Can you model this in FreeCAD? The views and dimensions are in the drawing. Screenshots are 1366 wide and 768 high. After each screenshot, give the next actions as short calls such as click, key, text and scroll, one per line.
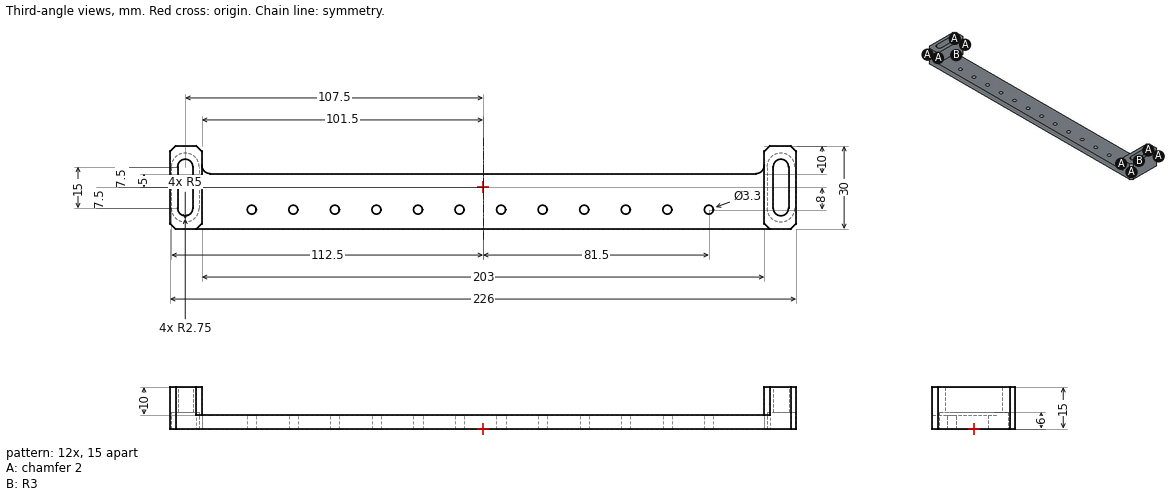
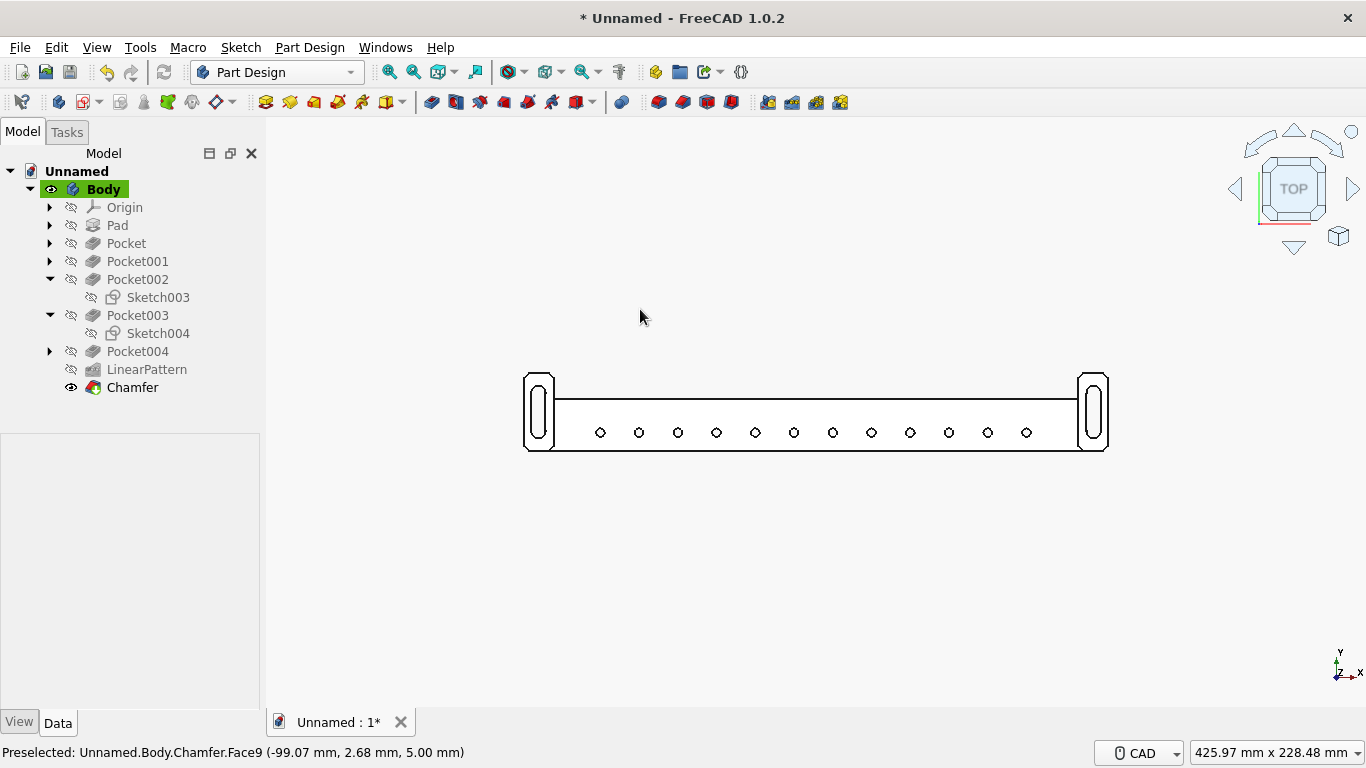
scroll(554, 398, up, 6)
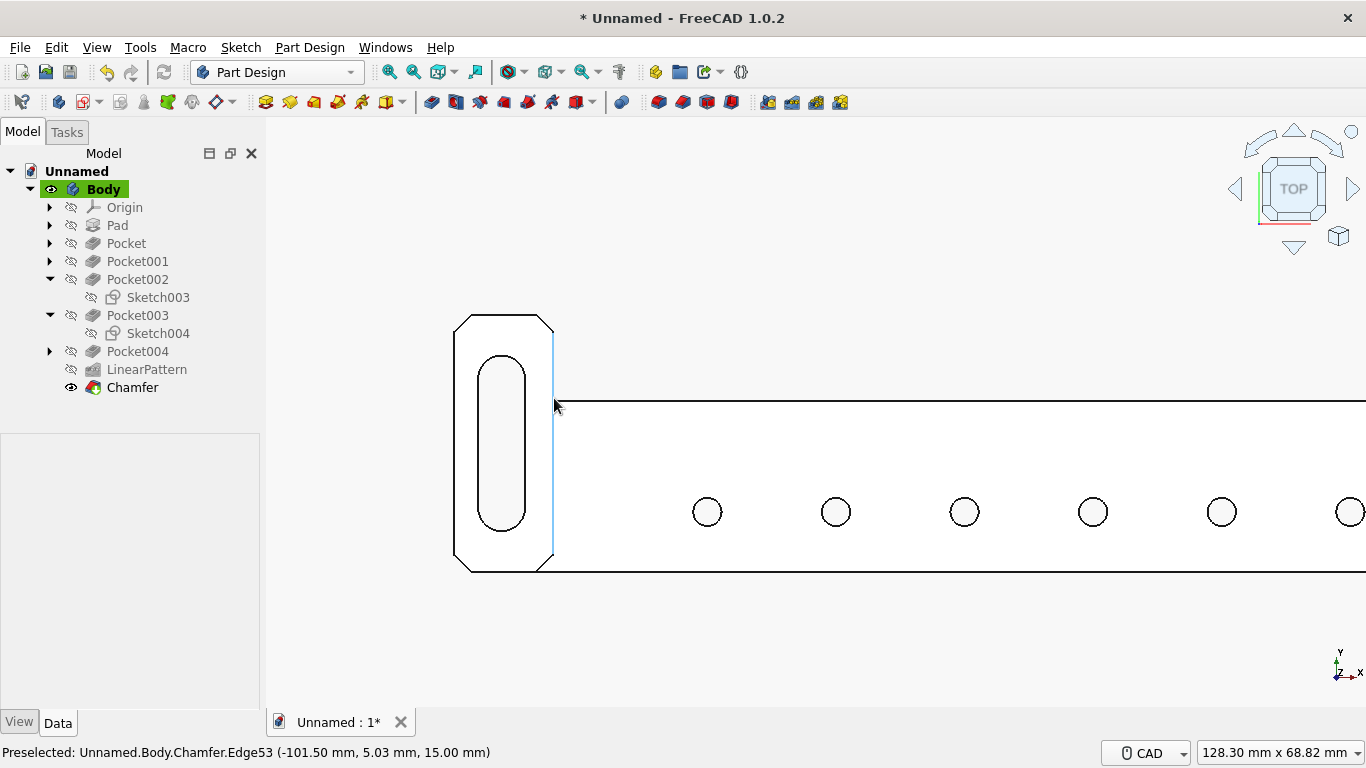
click(390, 72)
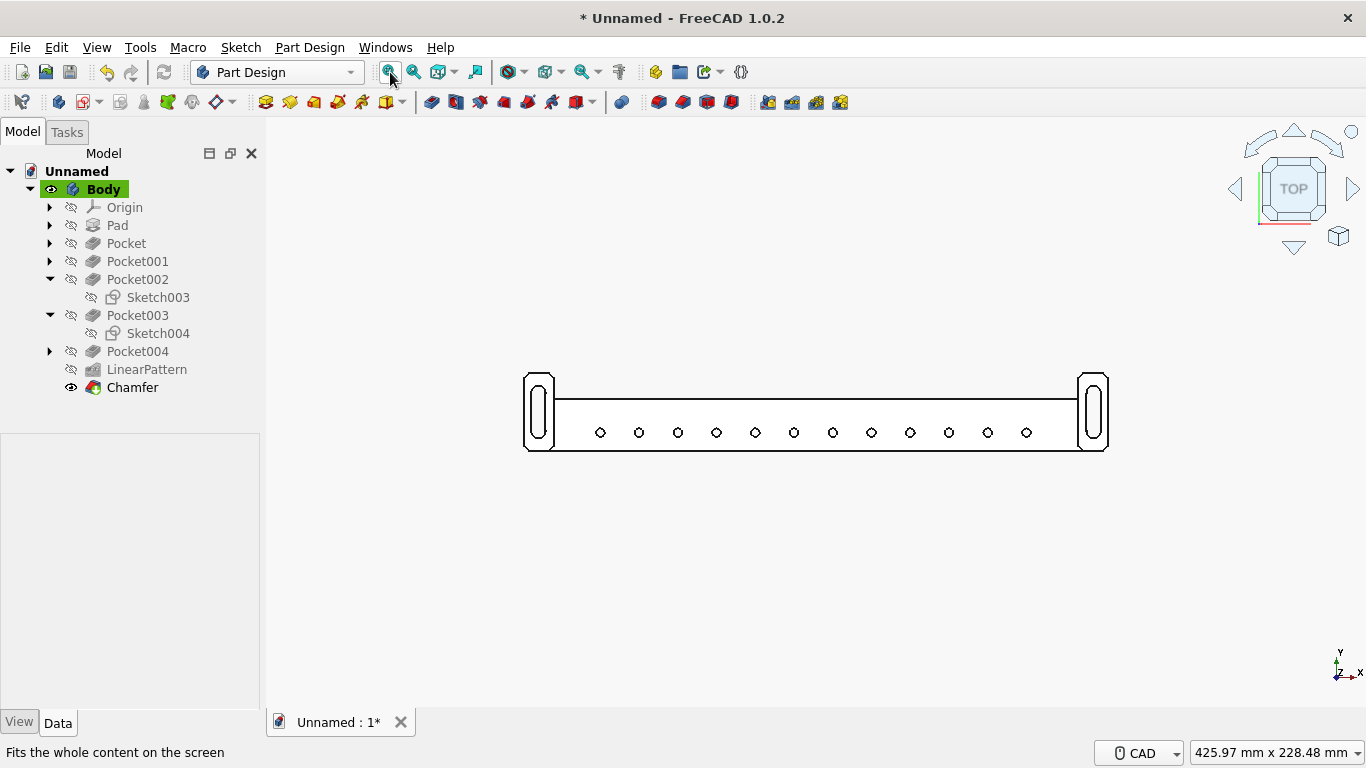
key(1)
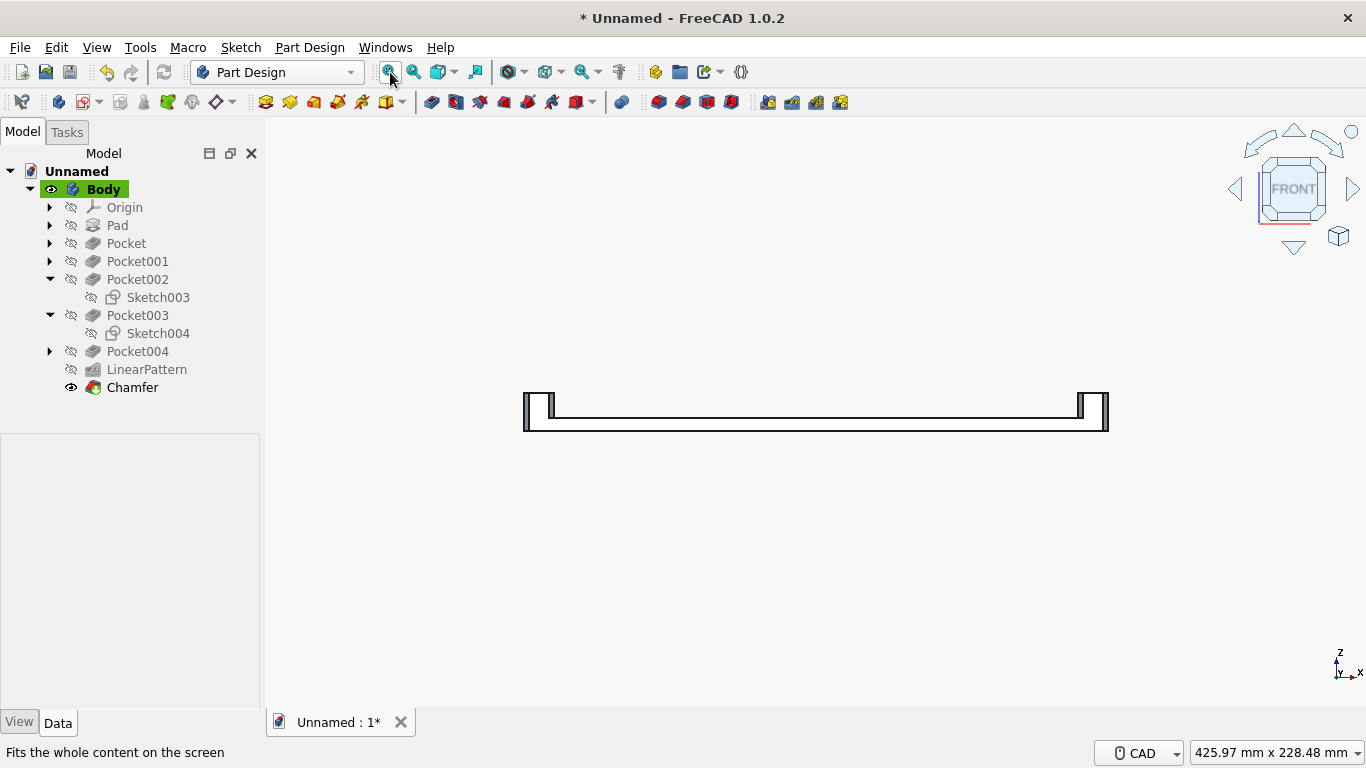
scroll(554, 424, up, 6)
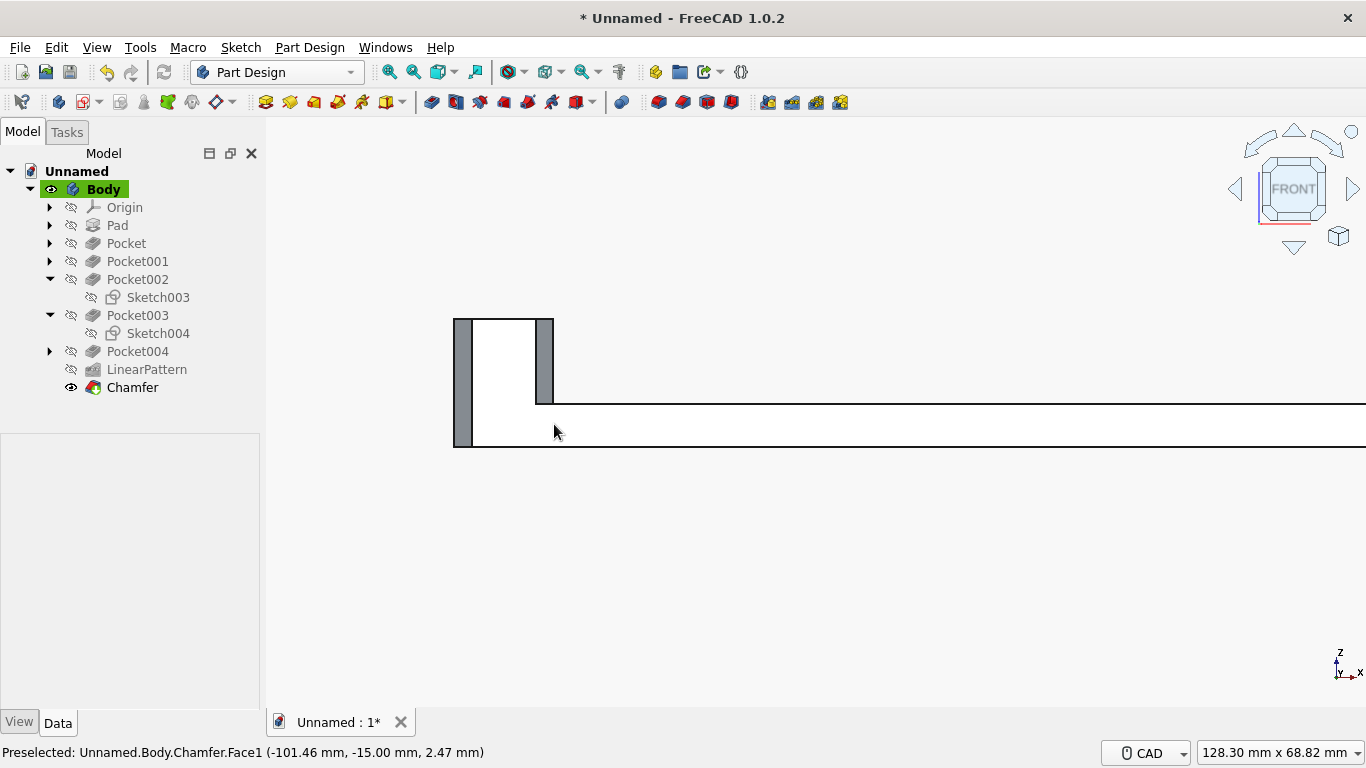
key(v)
key(f)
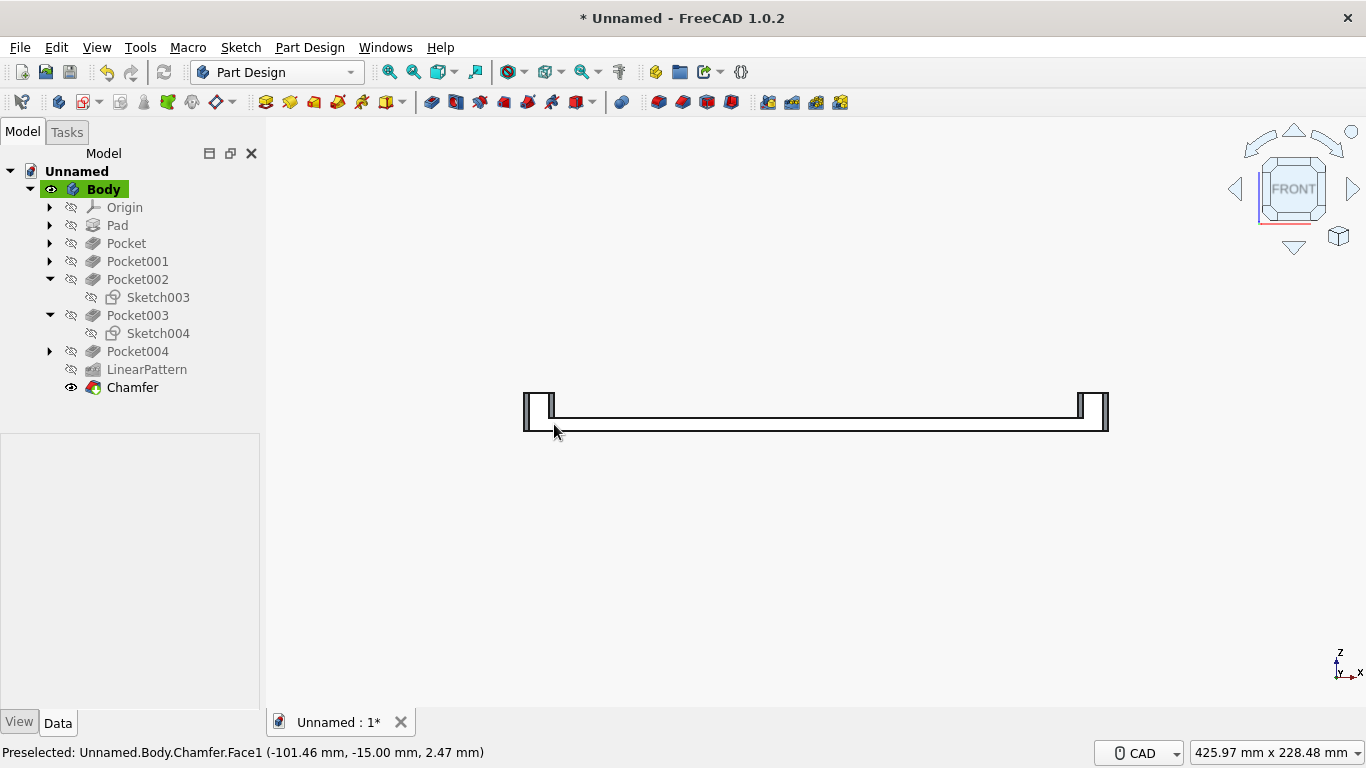
key(3)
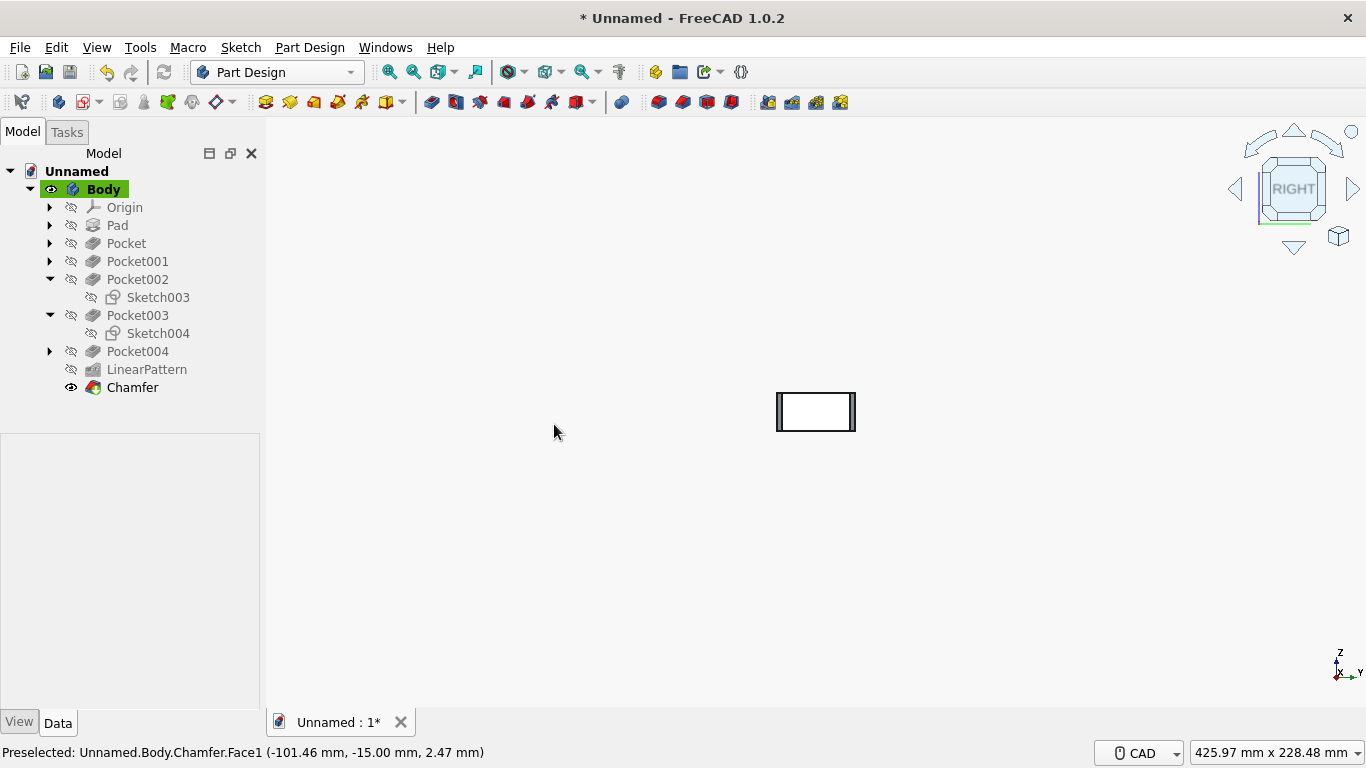
key(v)
key(f)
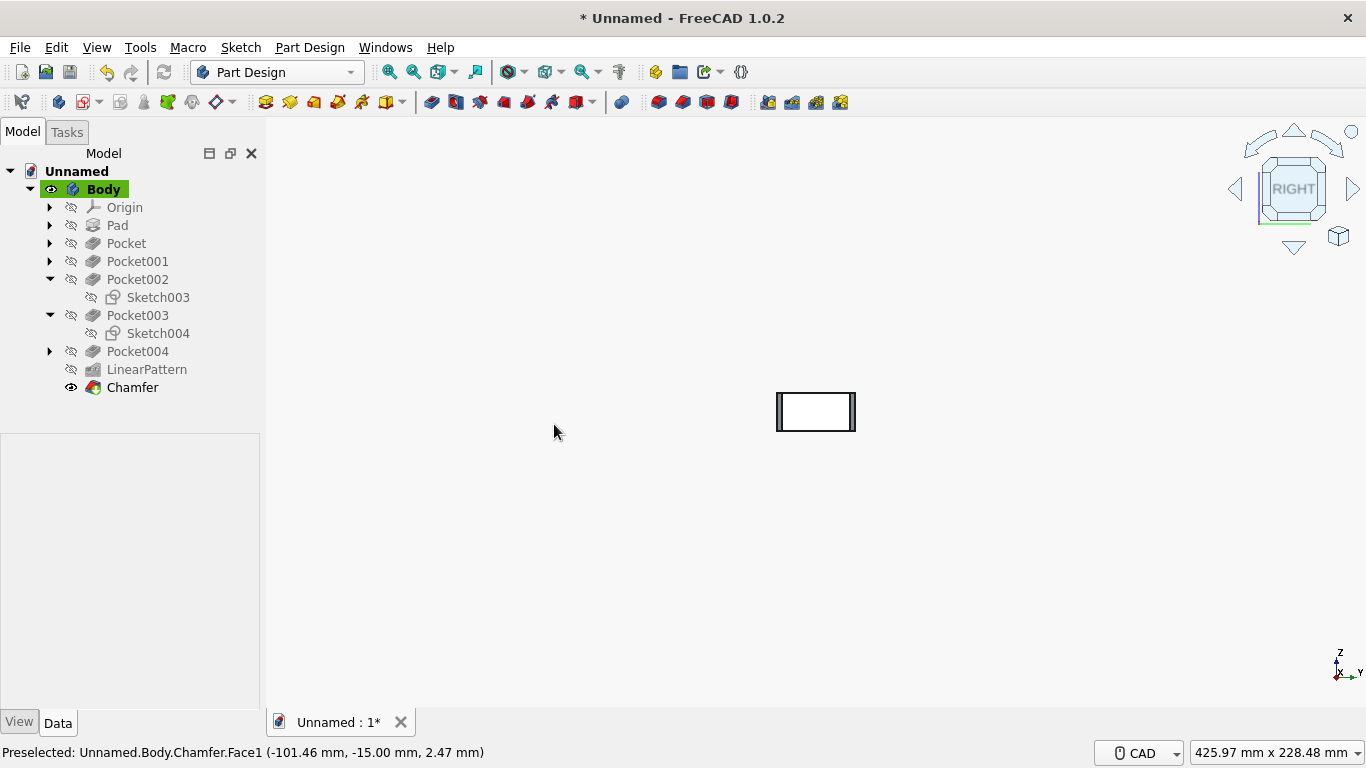
scroll(829, 424, up, 6)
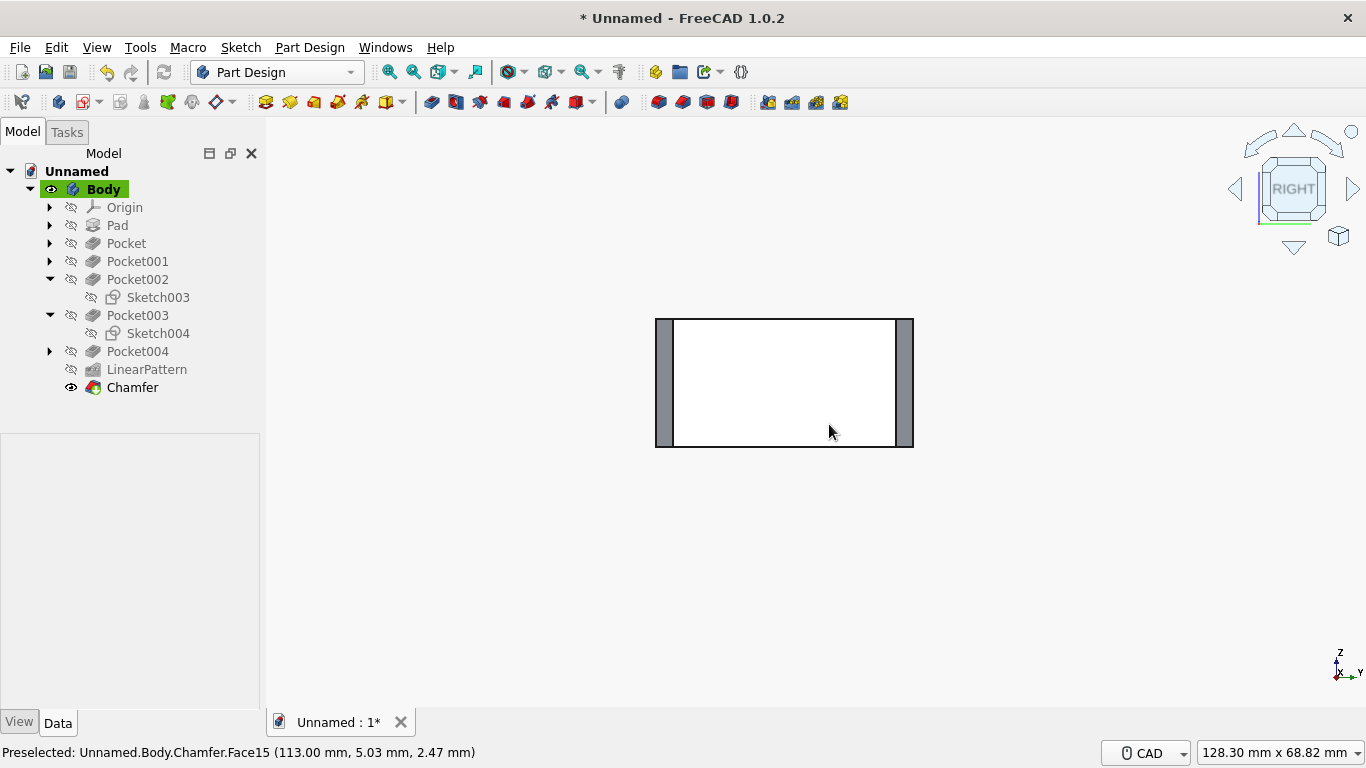
click(390, 72)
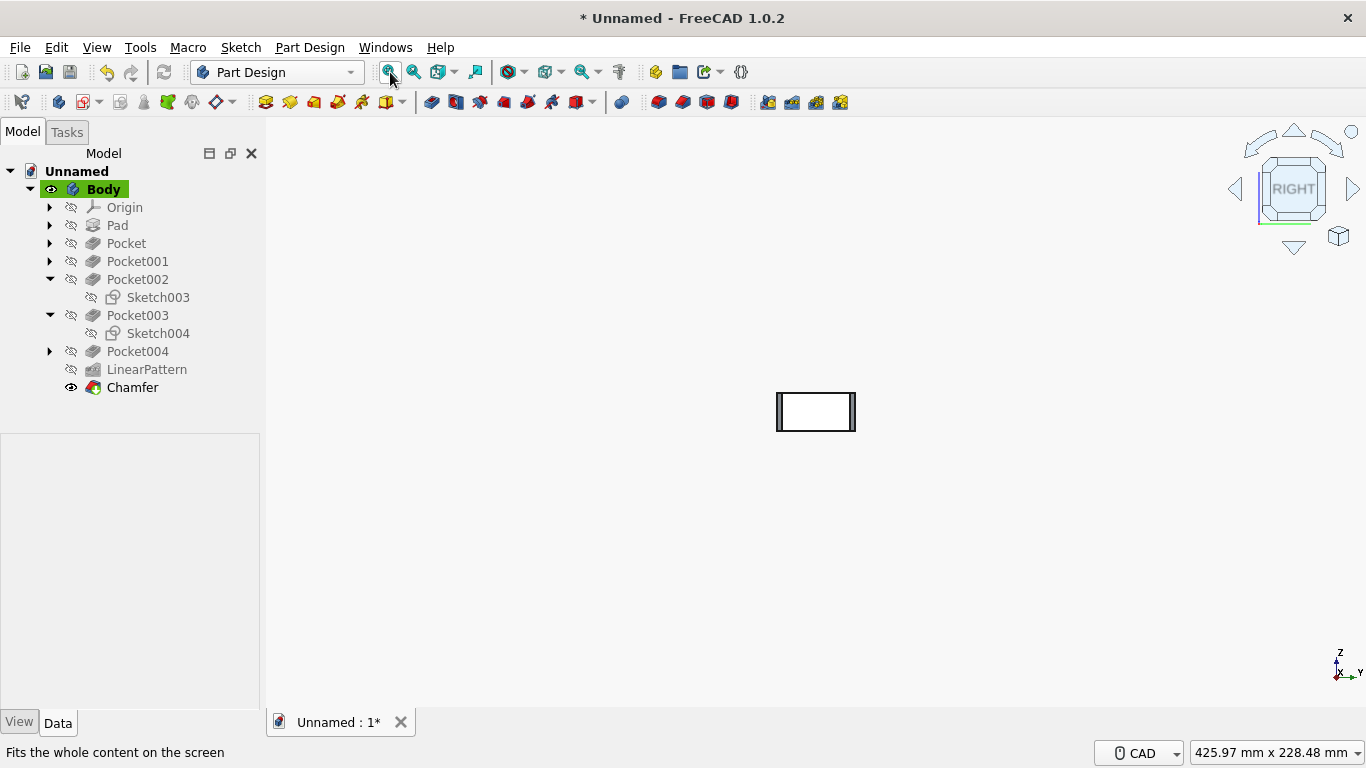
key(5)